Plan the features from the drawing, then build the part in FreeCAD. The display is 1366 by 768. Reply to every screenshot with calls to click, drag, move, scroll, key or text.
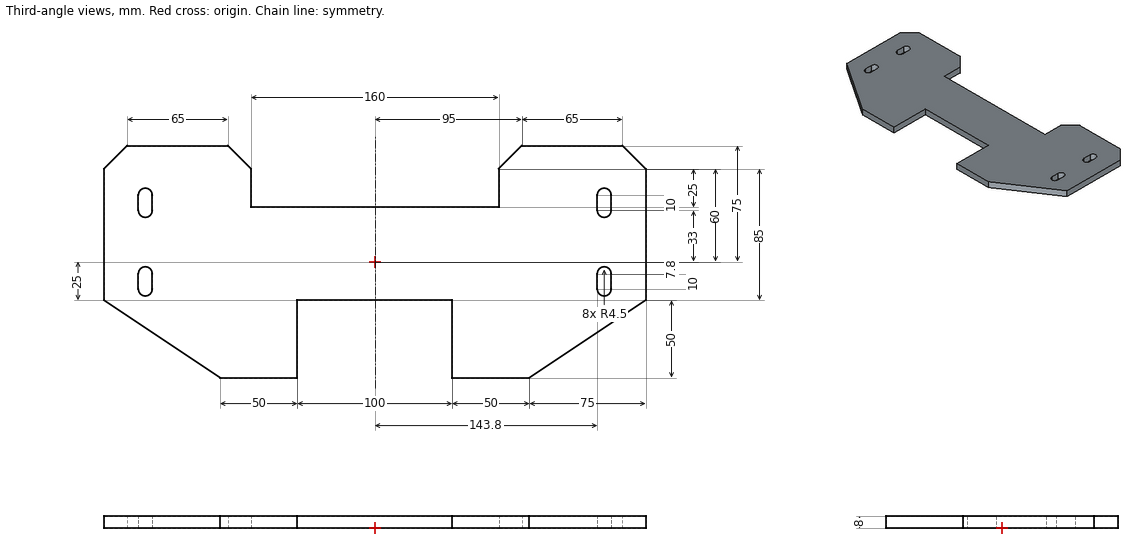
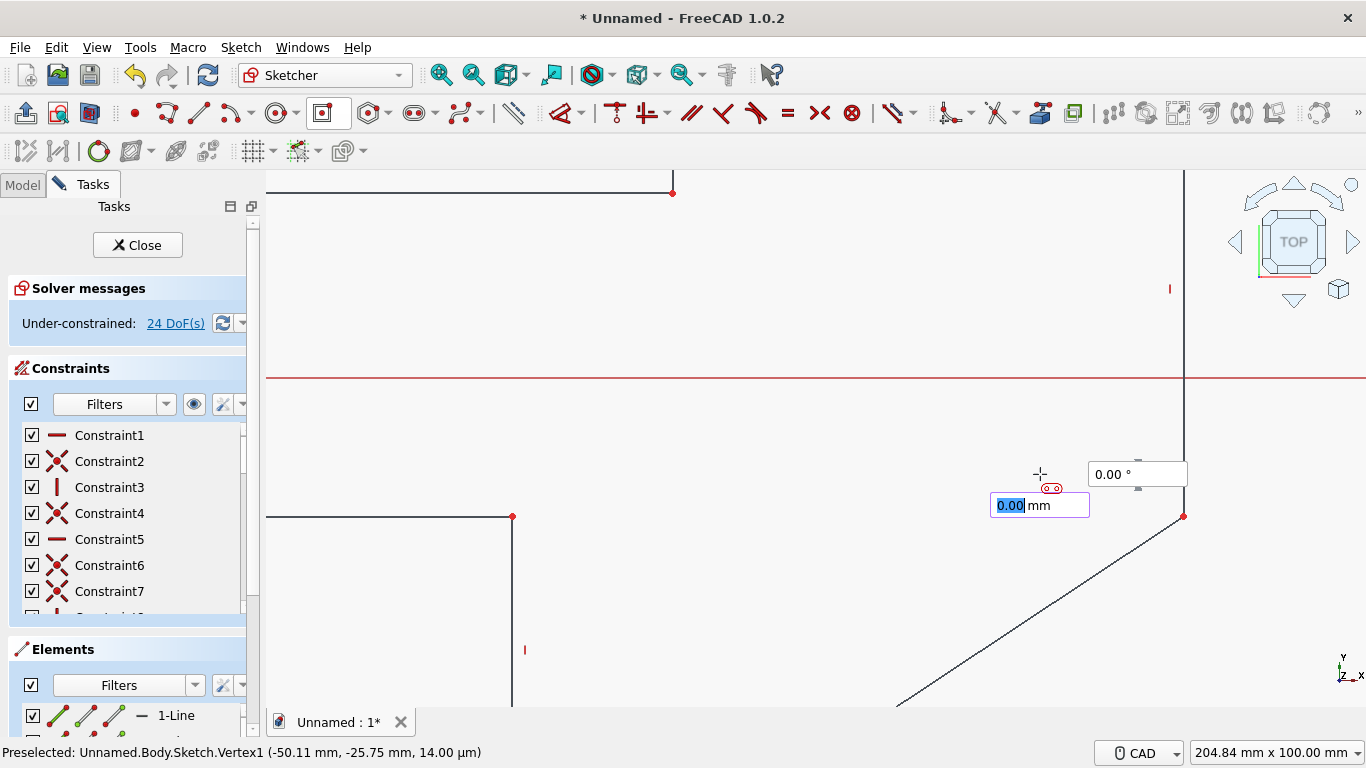
click(1040, 420)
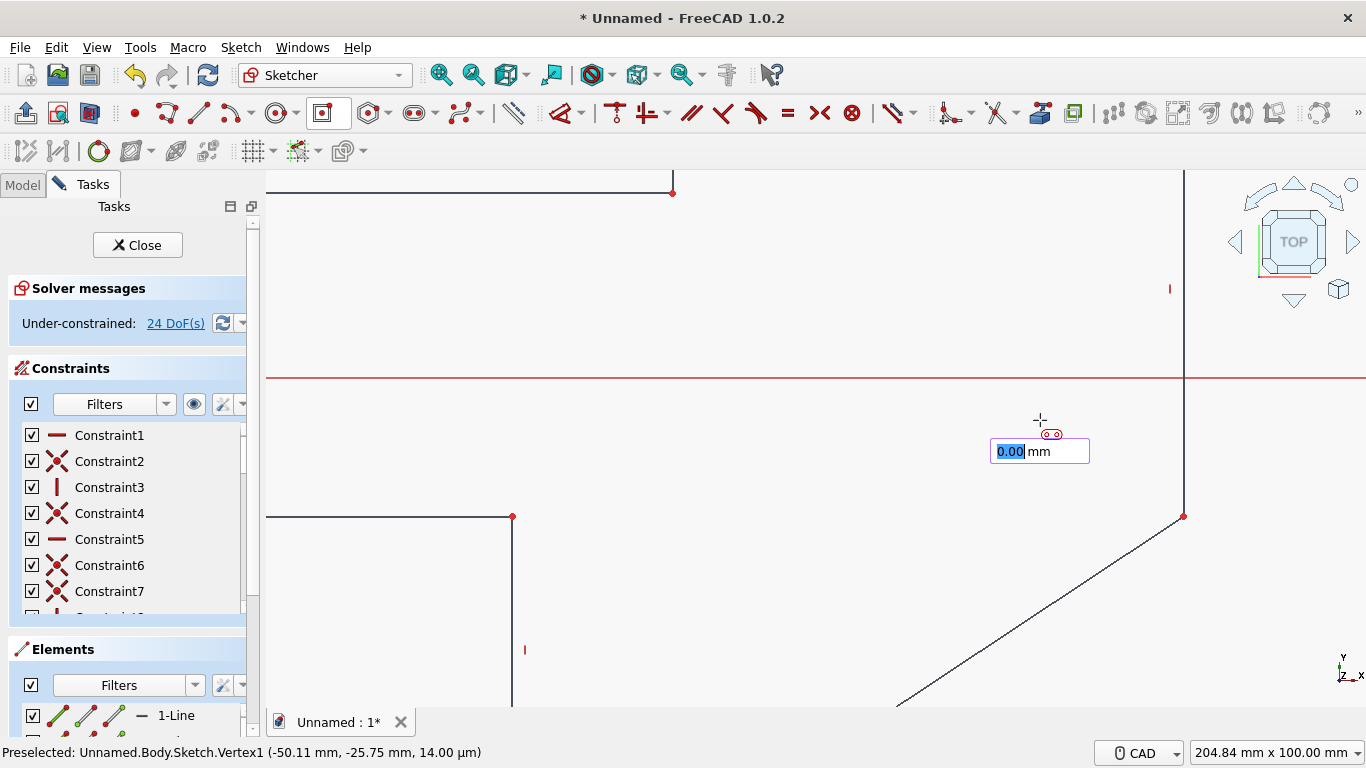
click(1064, 447)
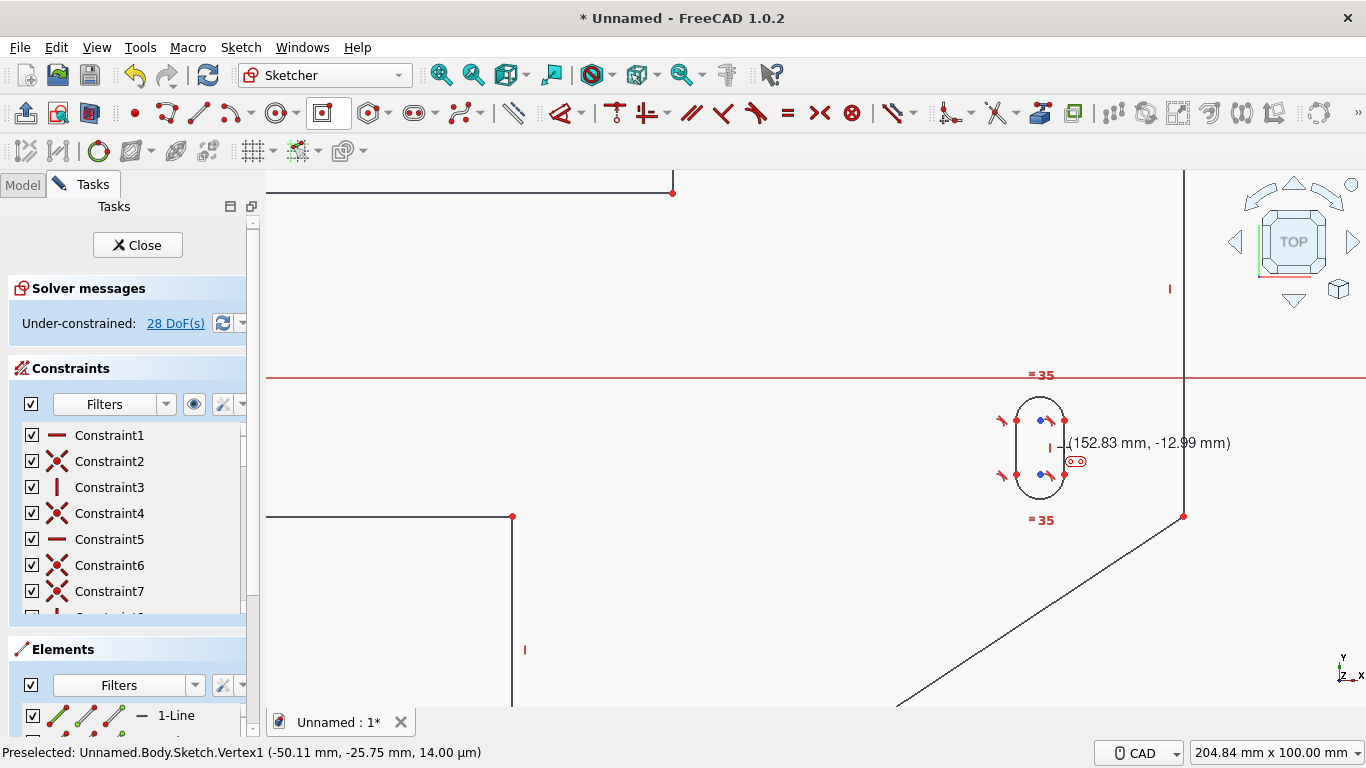
scroll(1041, 474, down, 5)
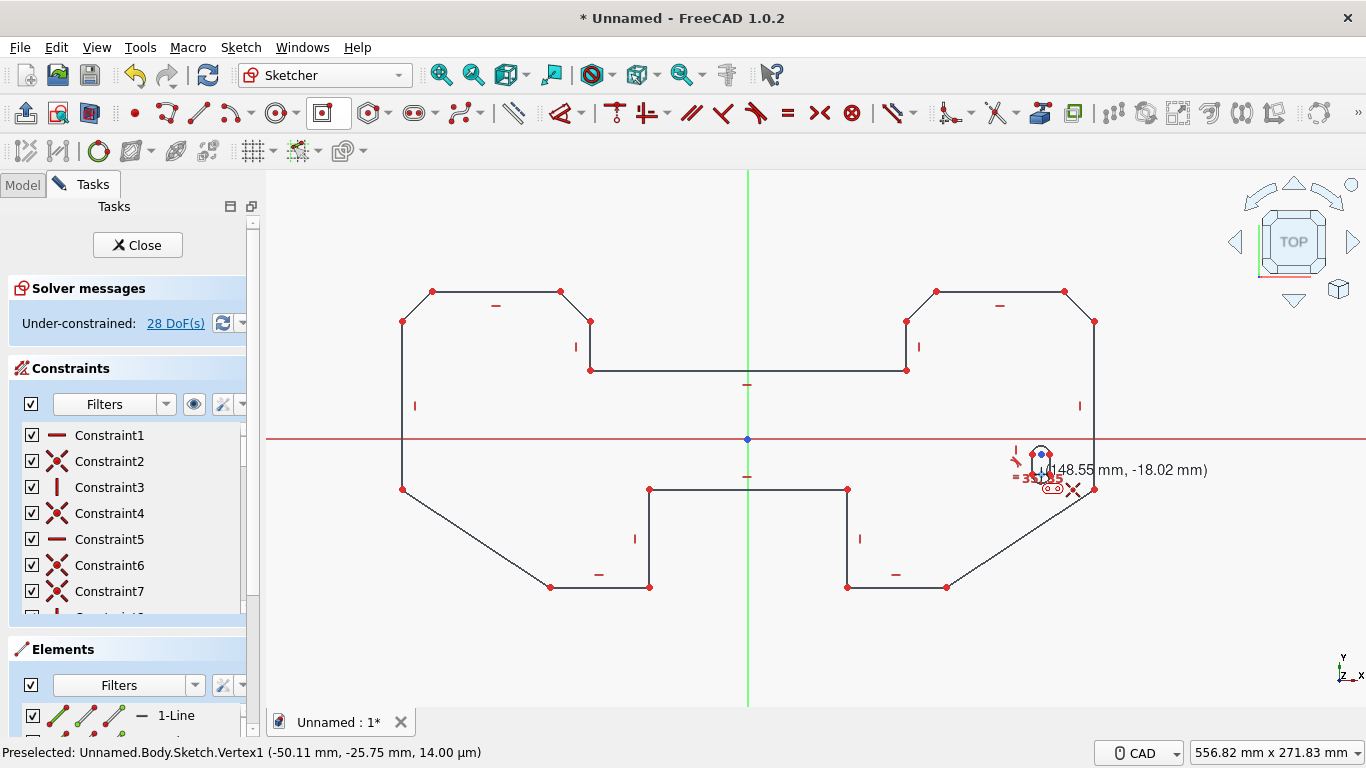
scroll(455, 474, up, 5)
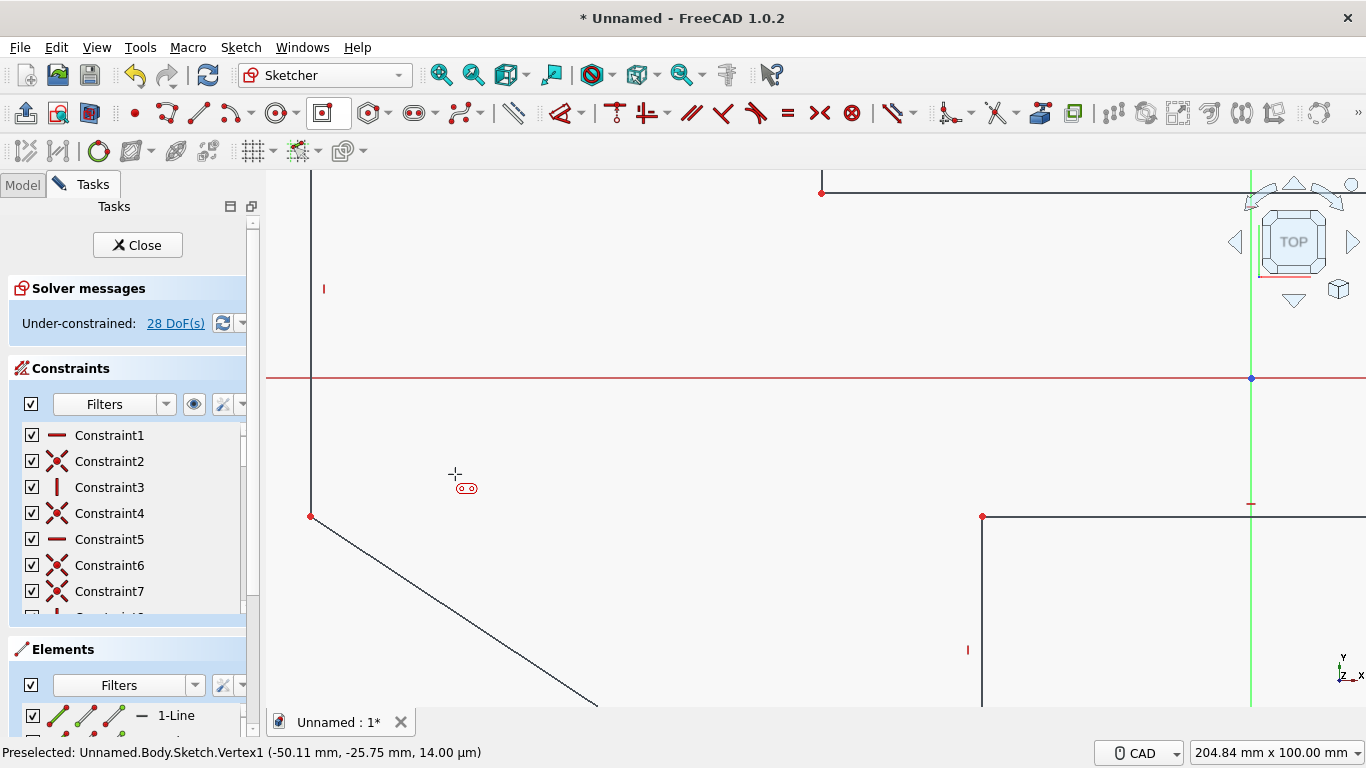
click(455, 474)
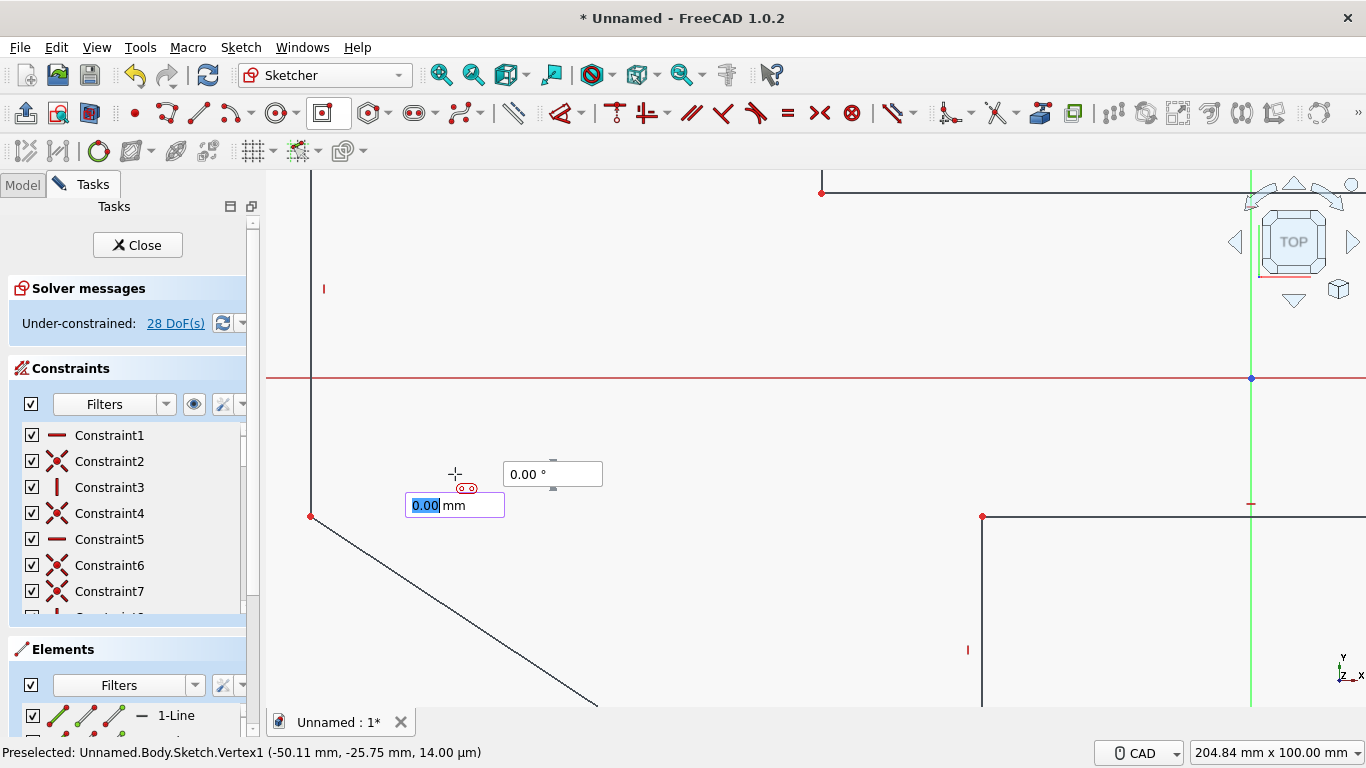
click(455, 420)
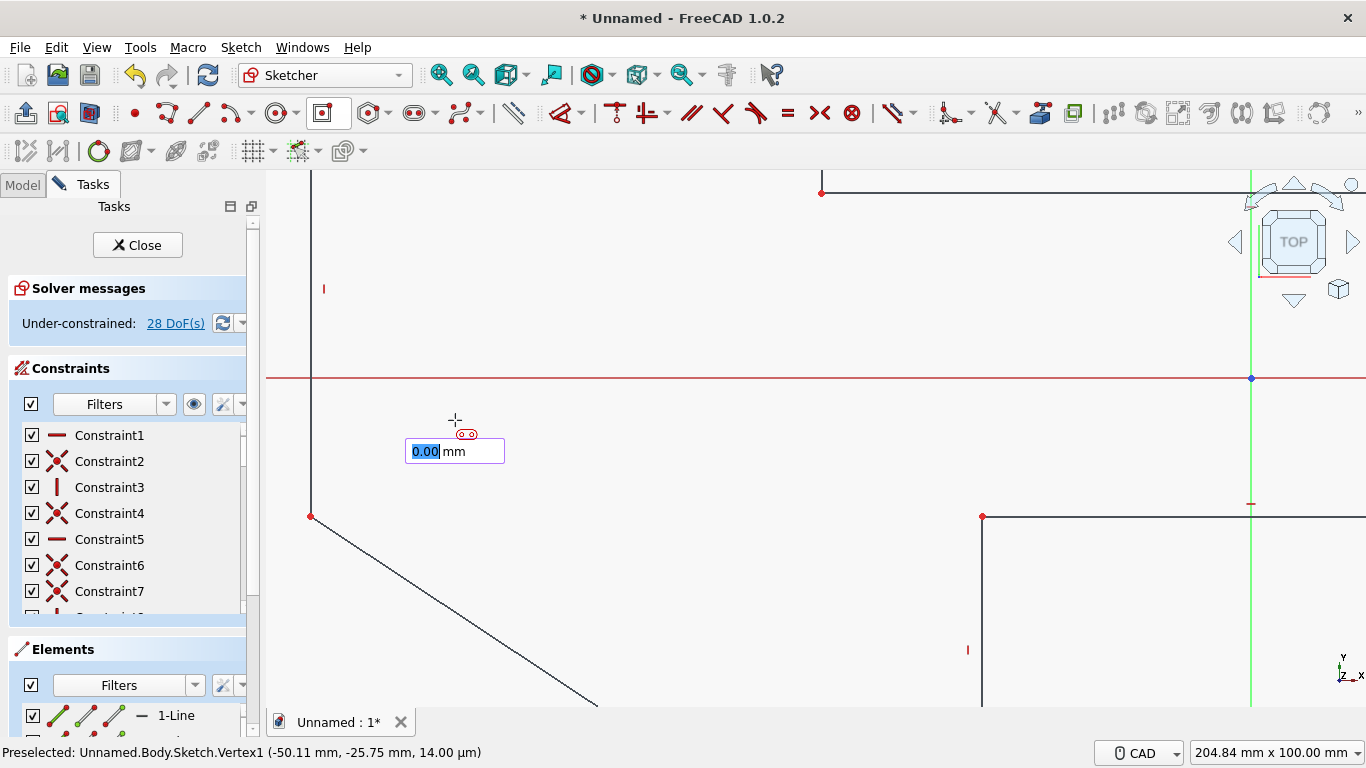
click(479, 447)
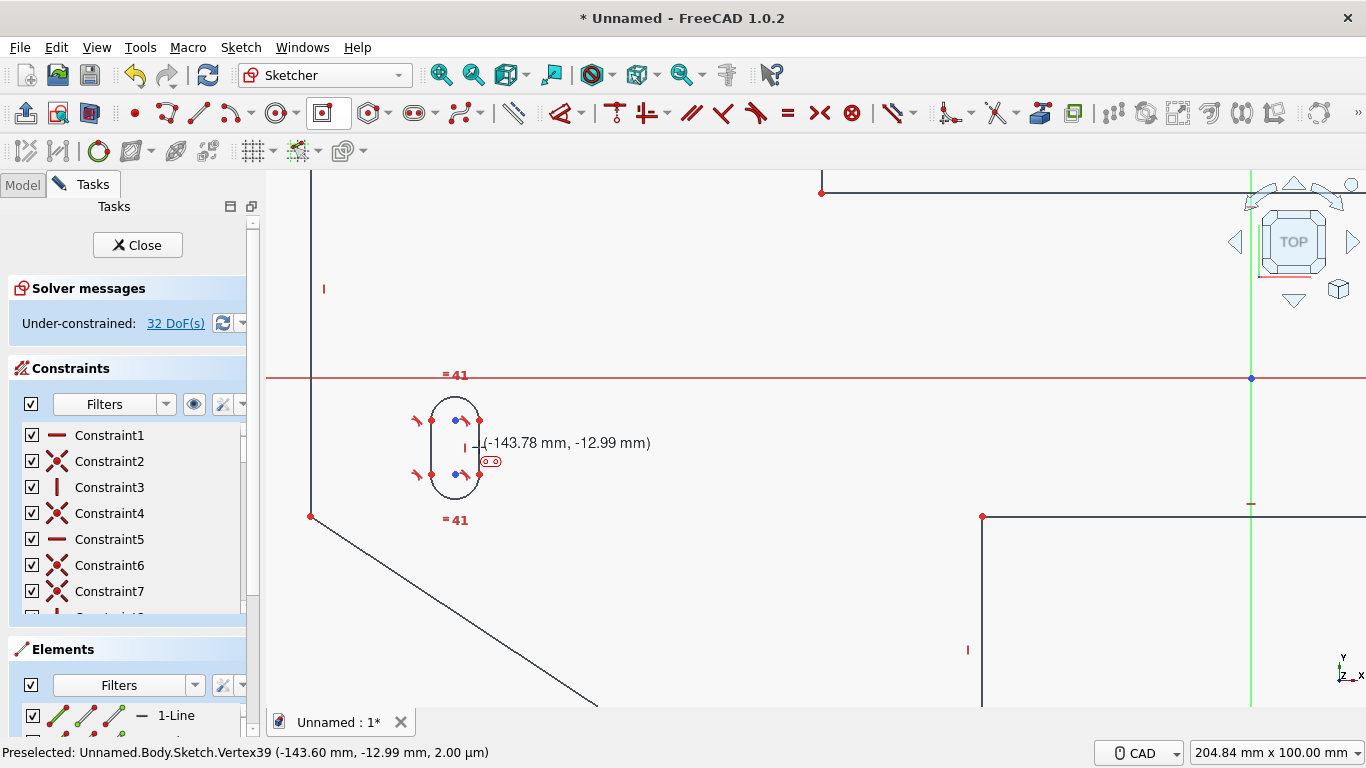
scroll(454, 474, down, 5)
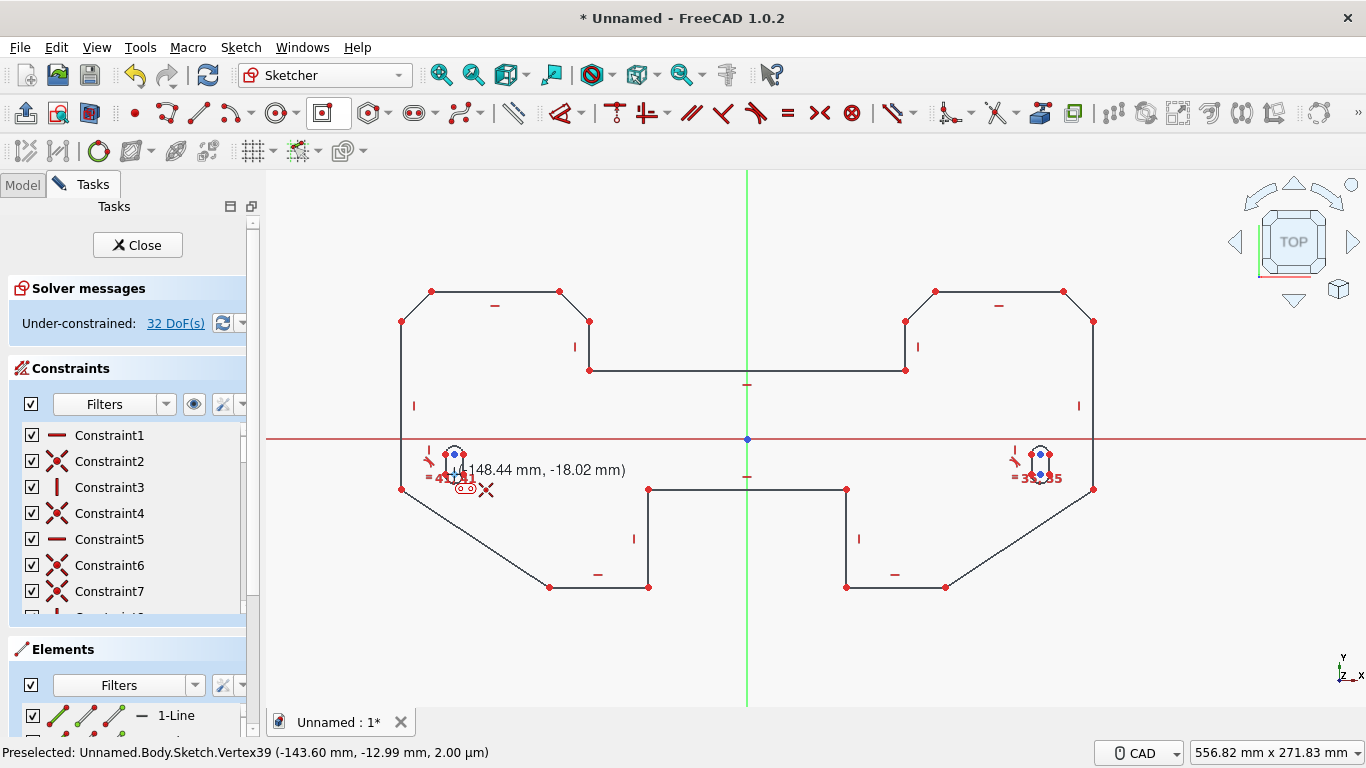
scroll(1040, 374, up, 5)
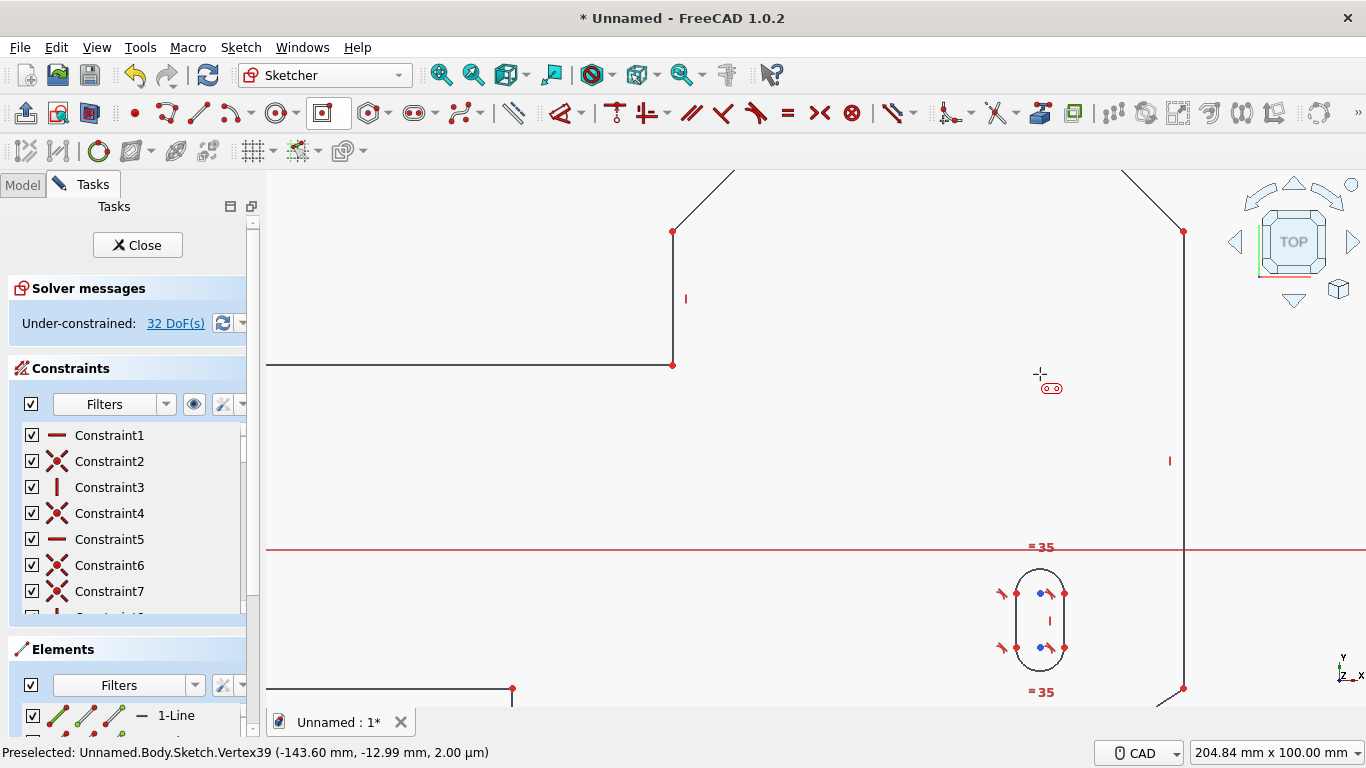
click(1040, 373)